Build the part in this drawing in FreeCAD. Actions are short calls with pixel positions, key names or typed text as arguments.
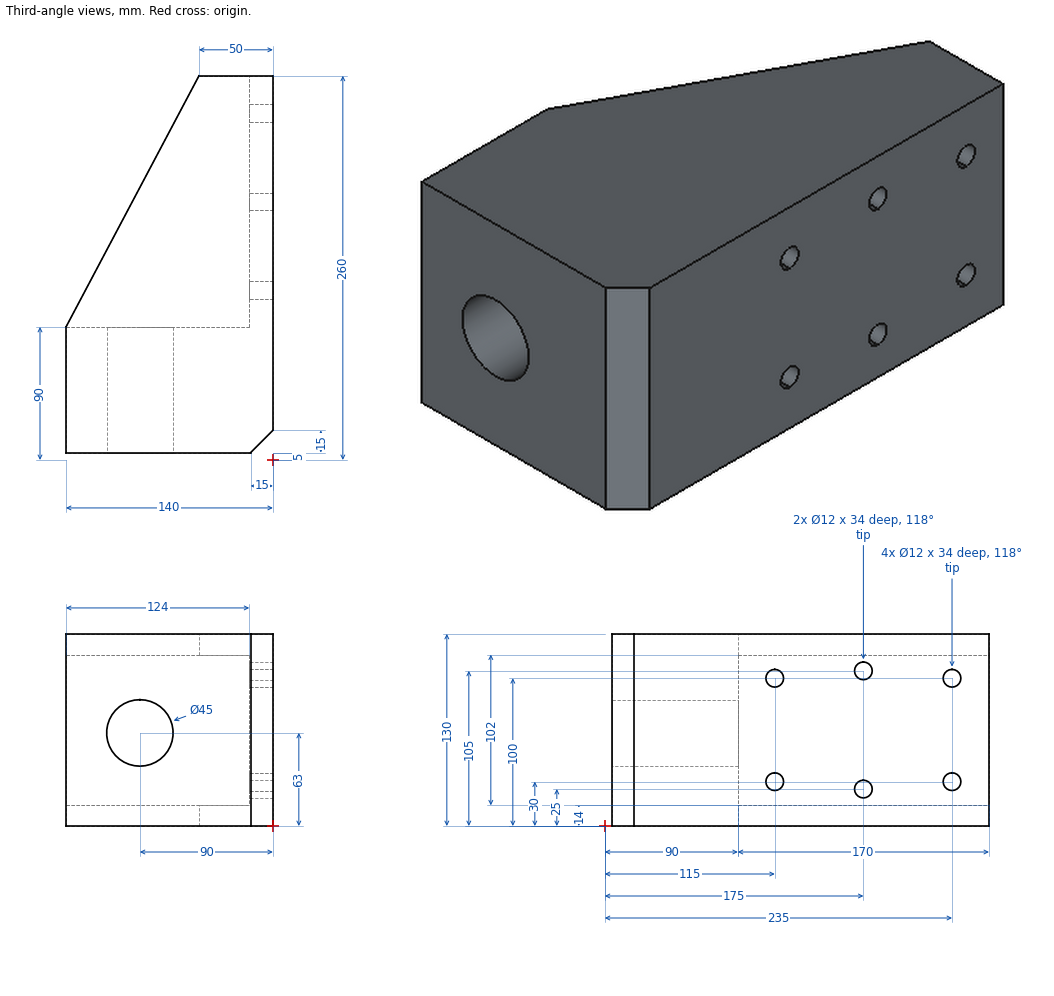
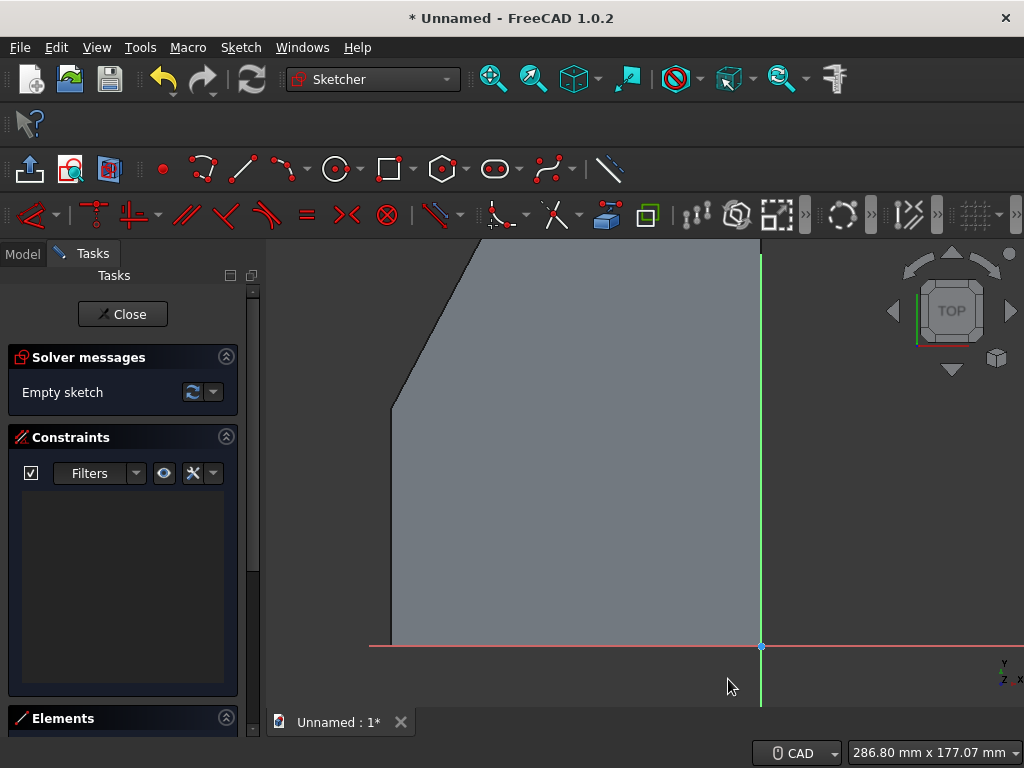
click(390, 170)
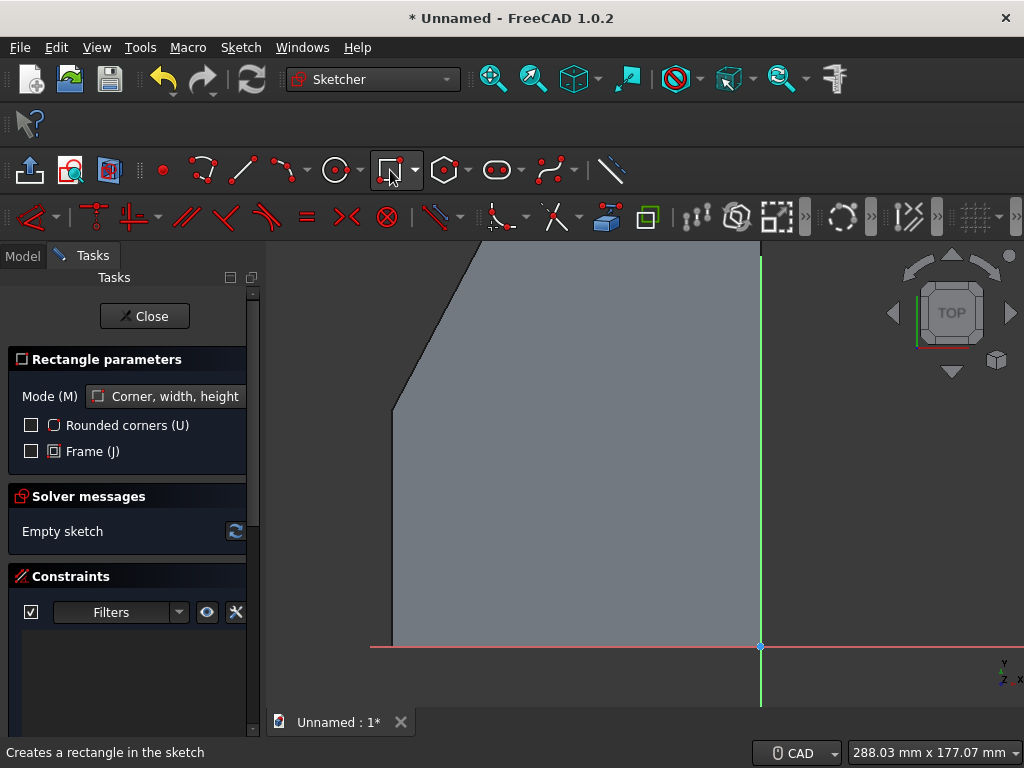
click(761, 647)
move(392, 634)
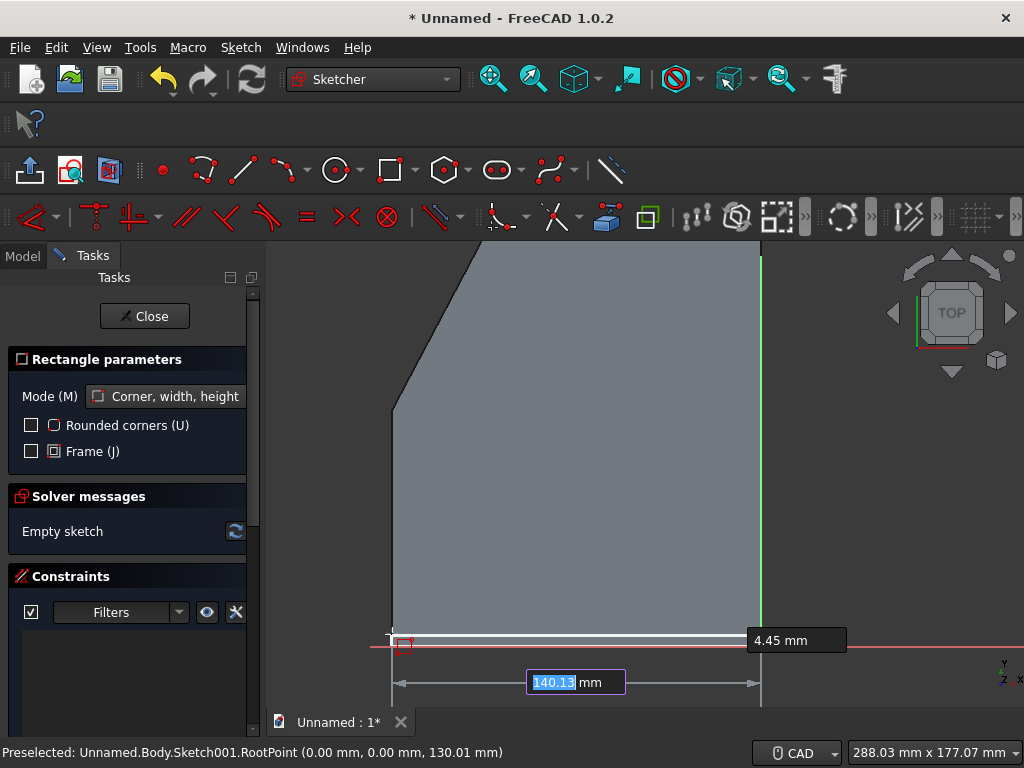
text(140)
key(Tab)
text(5)
key(Return)
key(Escape)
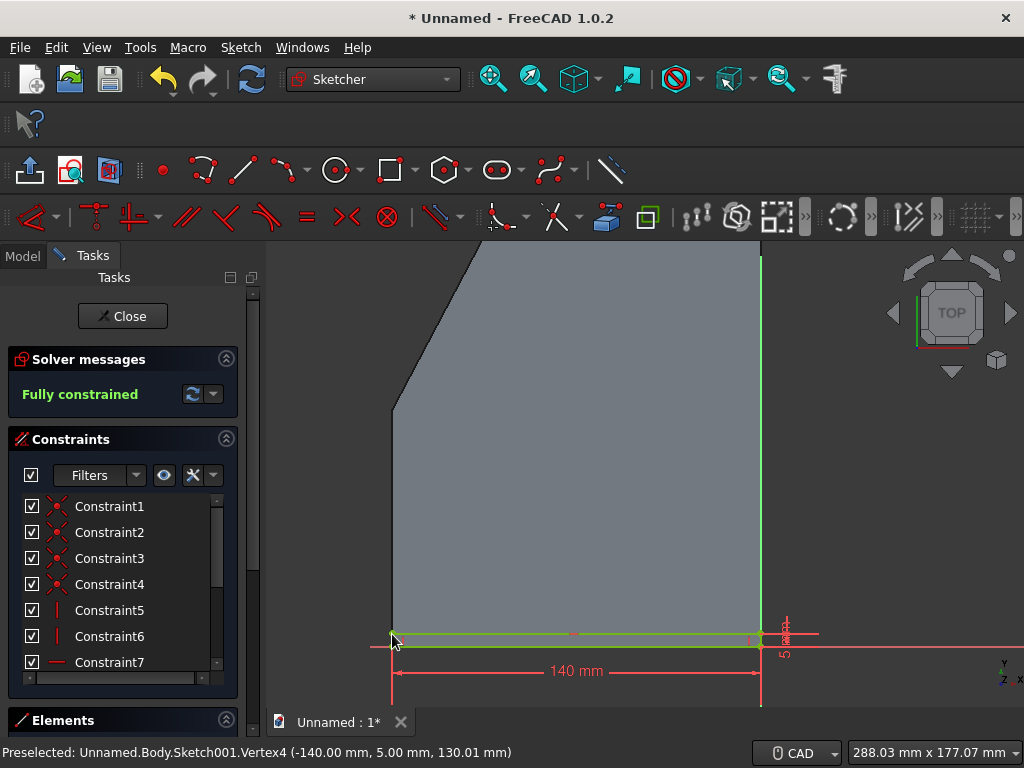
click(123, 316)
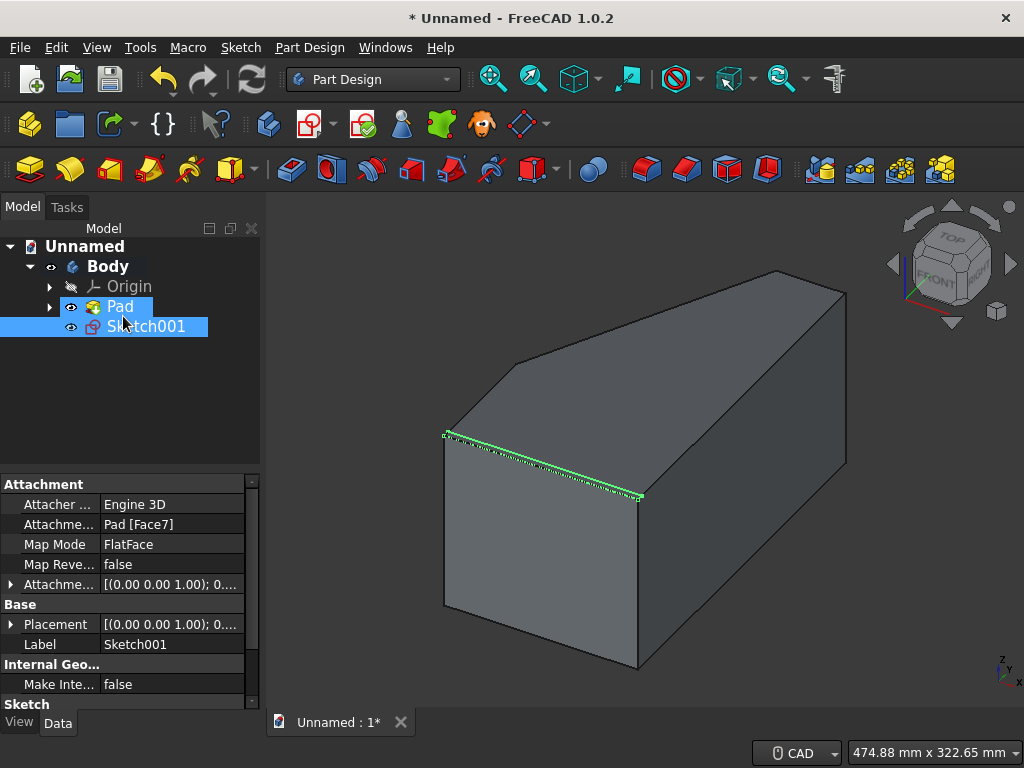
click(292, 170)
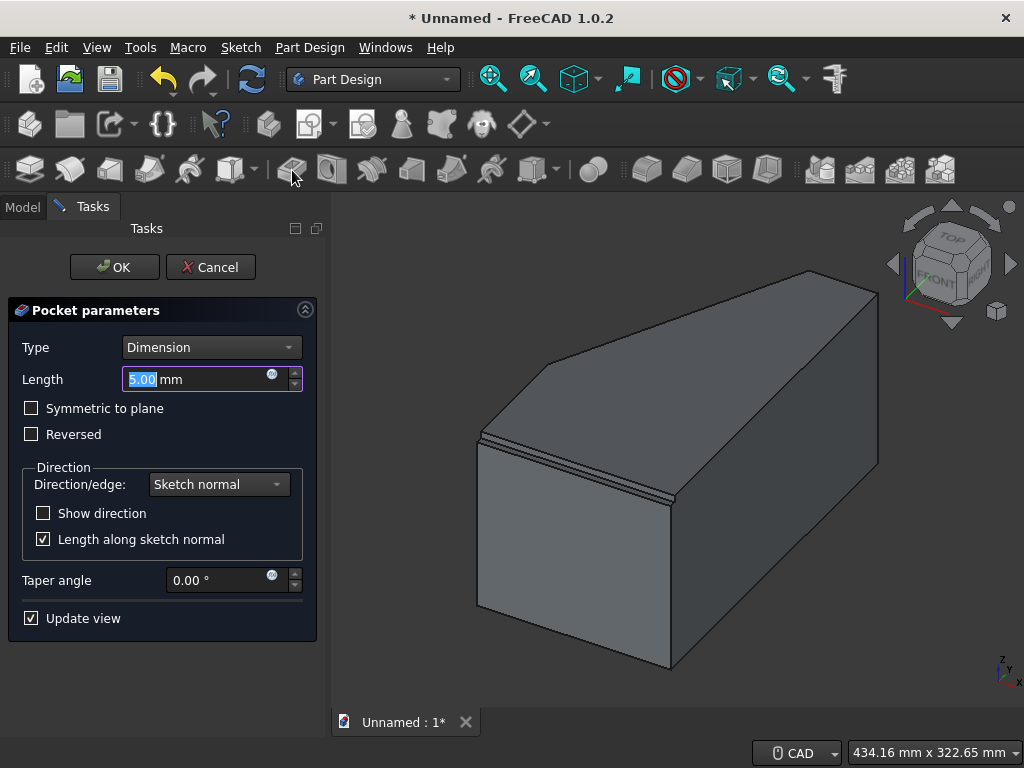
click(212, 348)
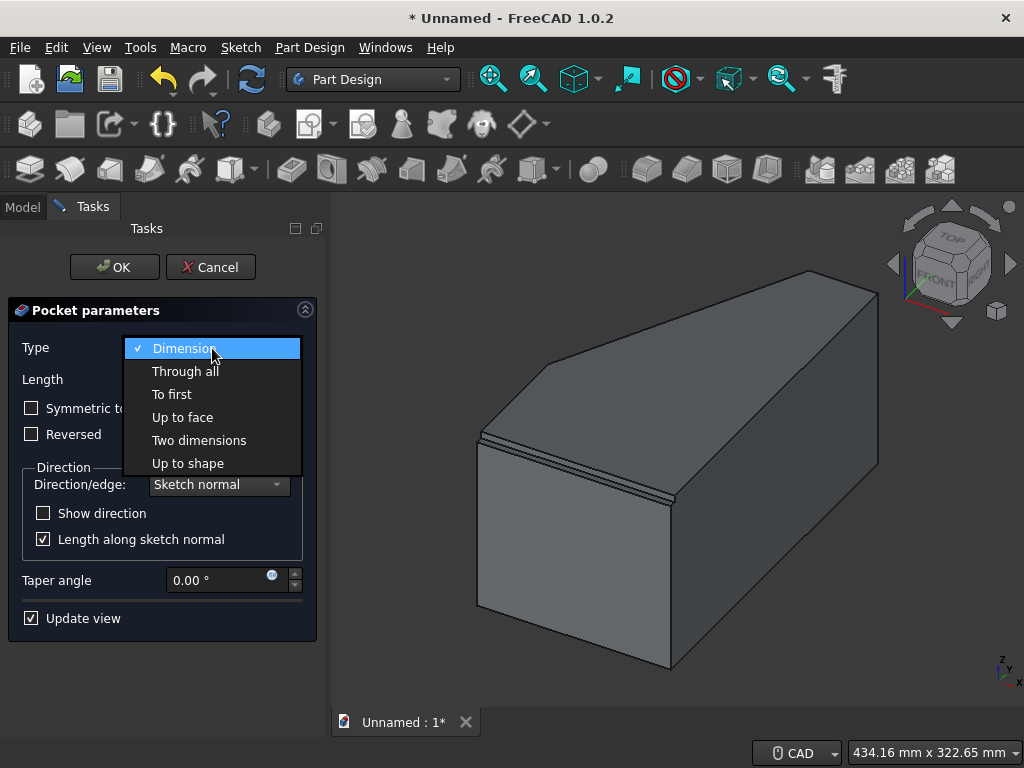
click(212, 372)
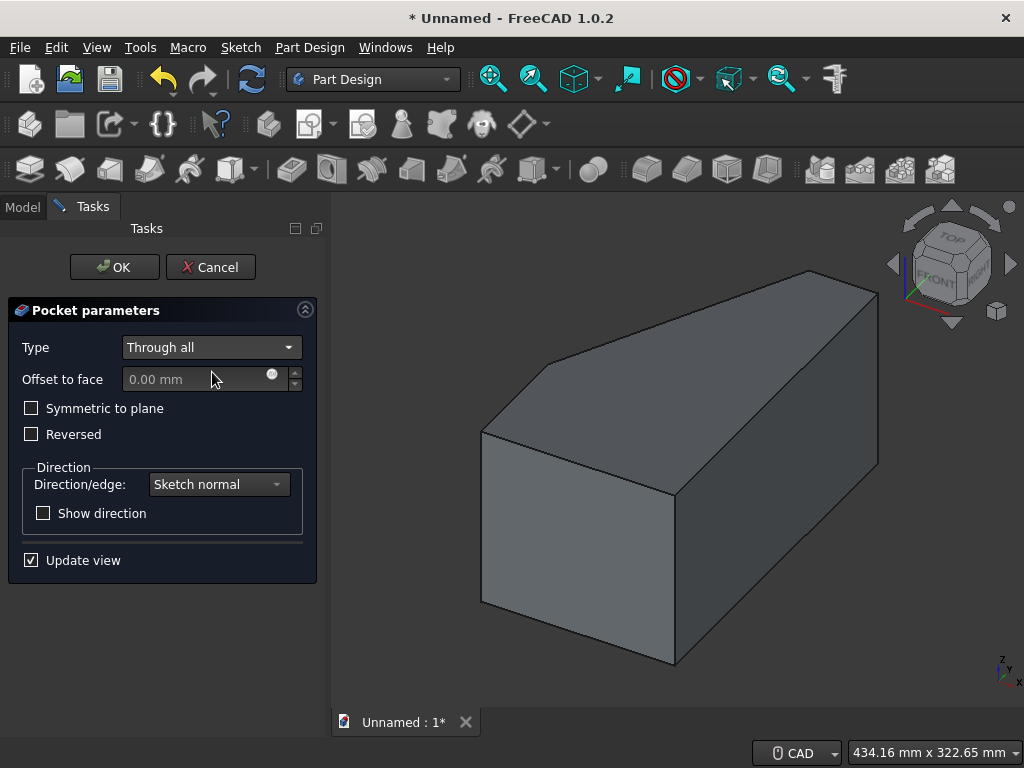
click(115, 267)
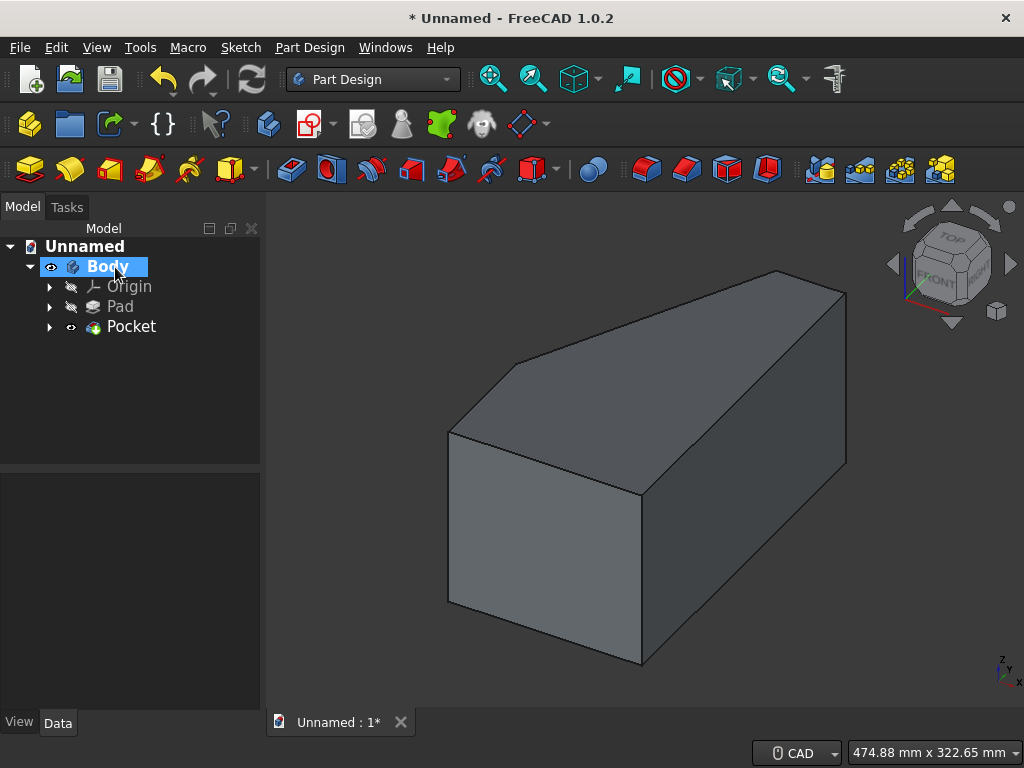
key(6)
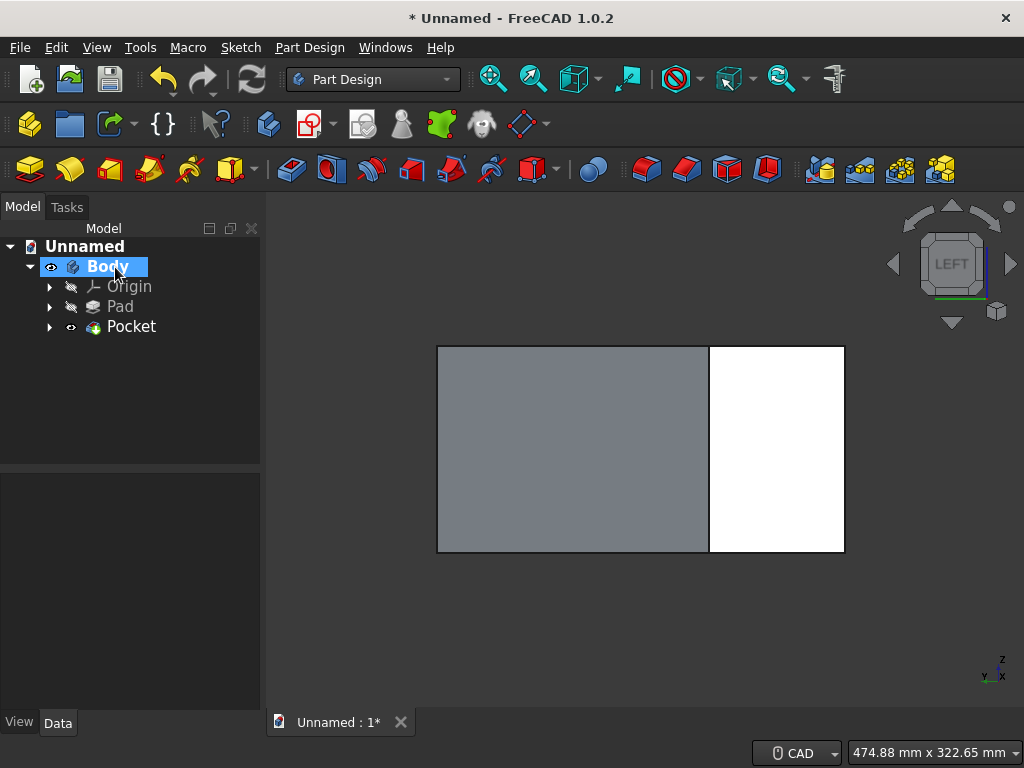
click(777, 419)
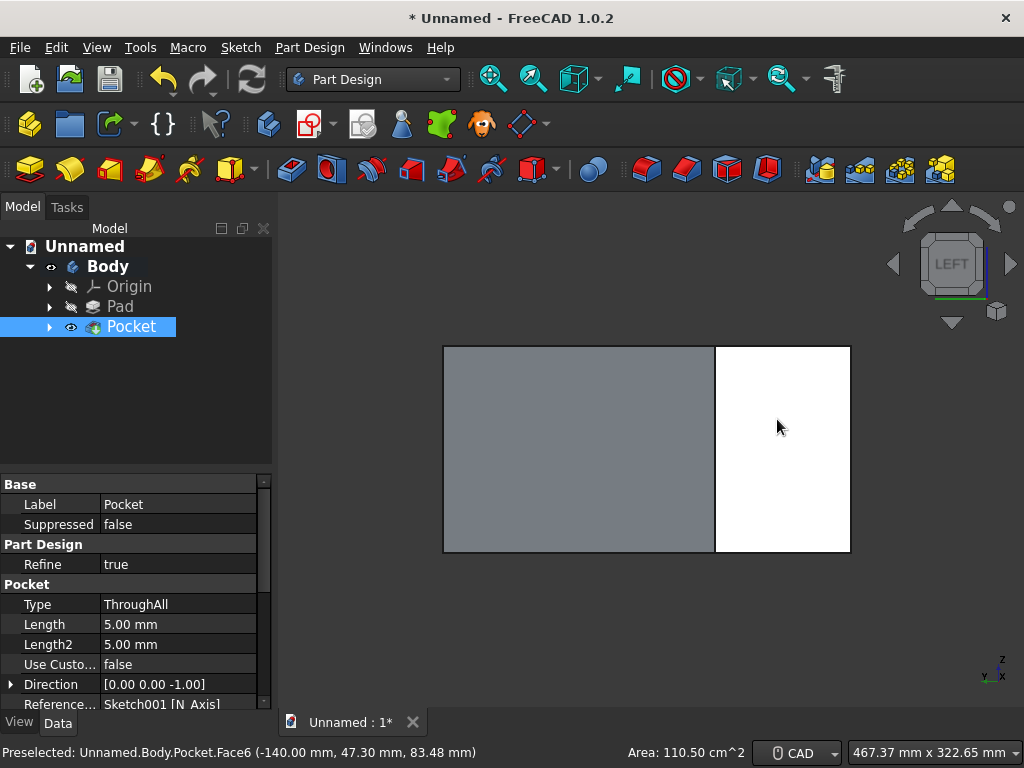
click(310, 124)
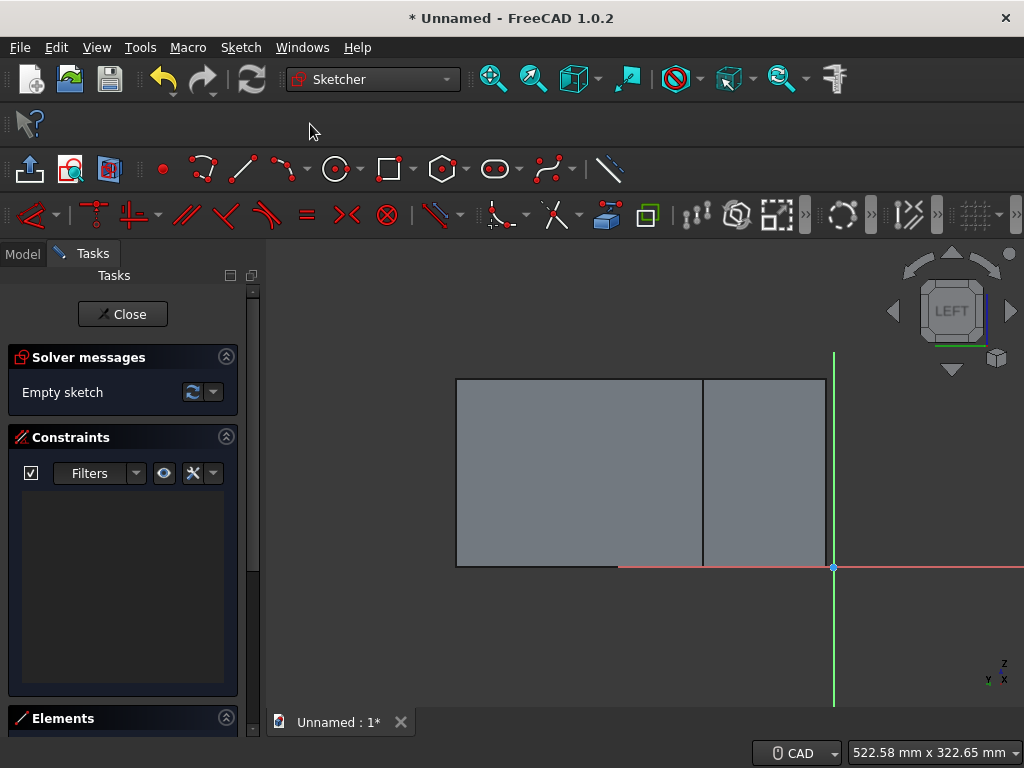
click(390, 170)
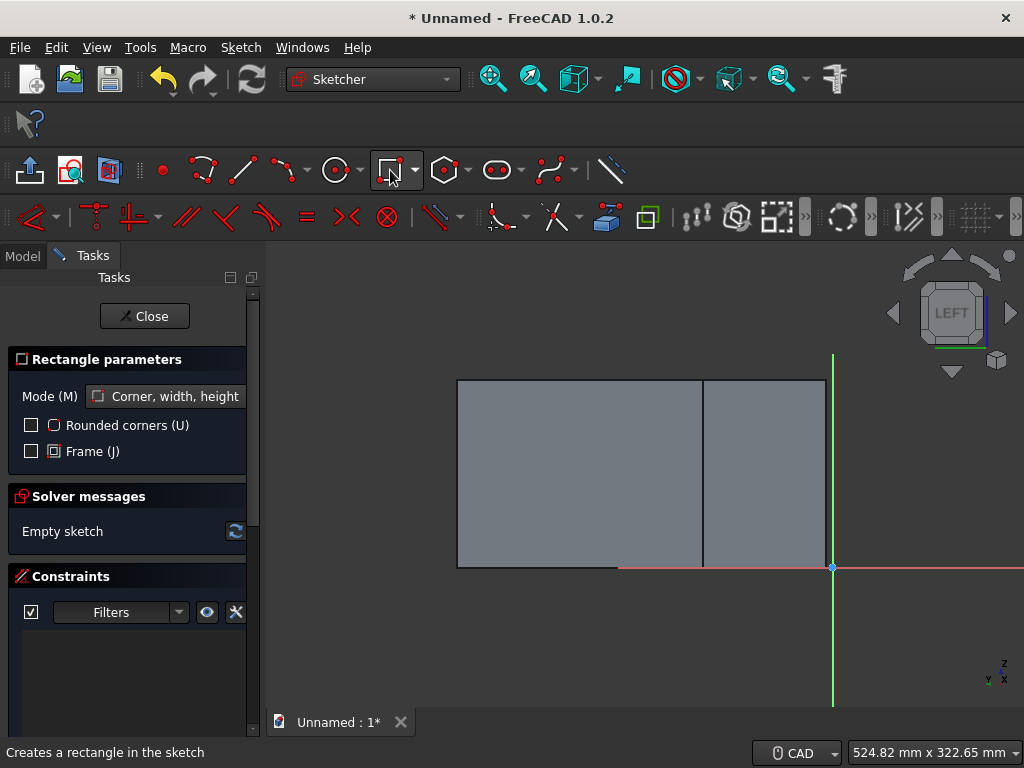
click(457, 400)
move(703, 548)